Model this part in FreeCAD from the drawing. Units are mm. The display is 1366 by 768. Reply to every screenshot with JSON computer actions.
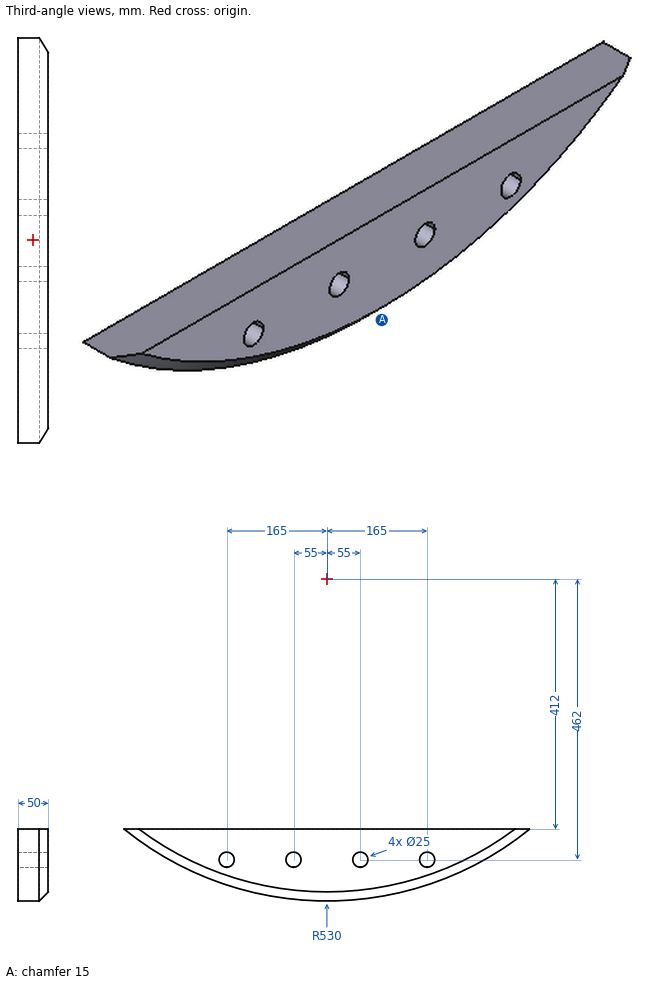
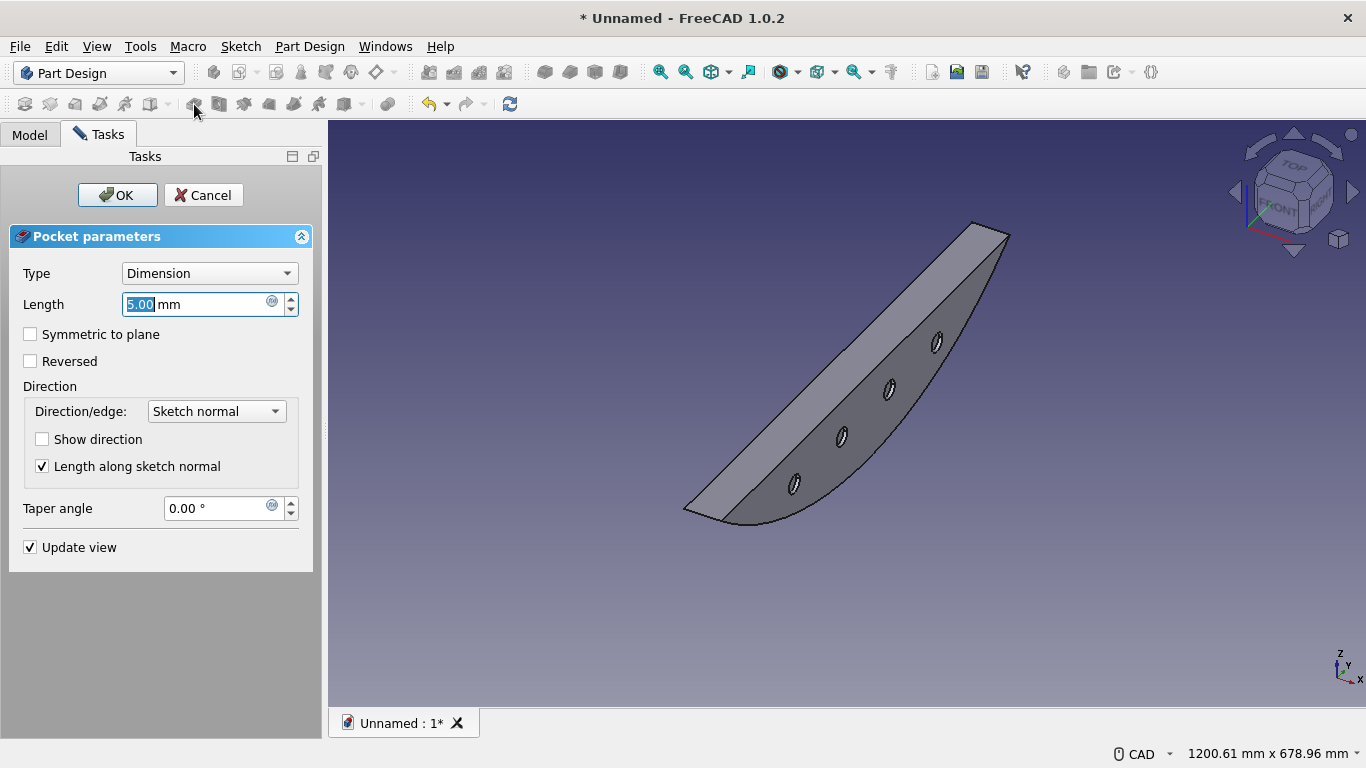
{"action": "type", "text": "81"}
{"action": "key", "text": "Tab"}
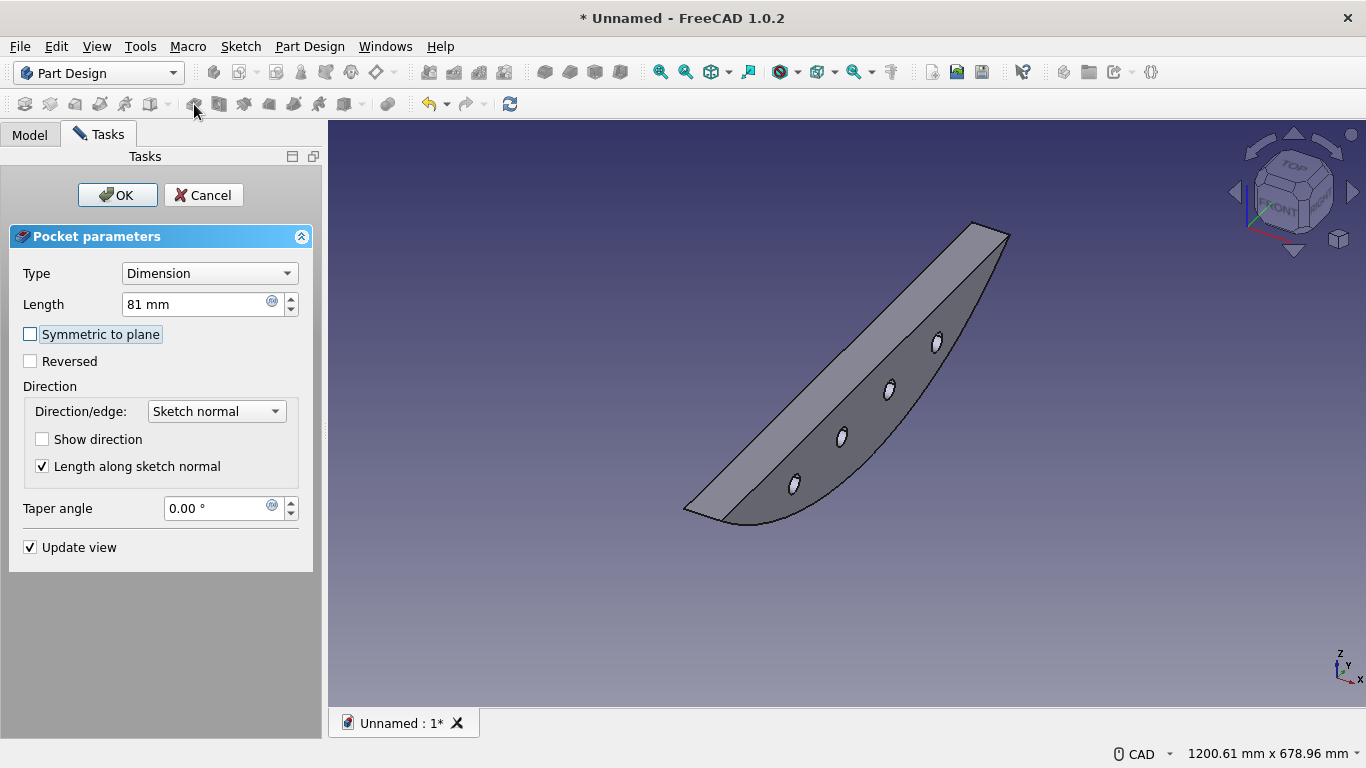
{"action": "left_click", "coordinate": [118, 195]}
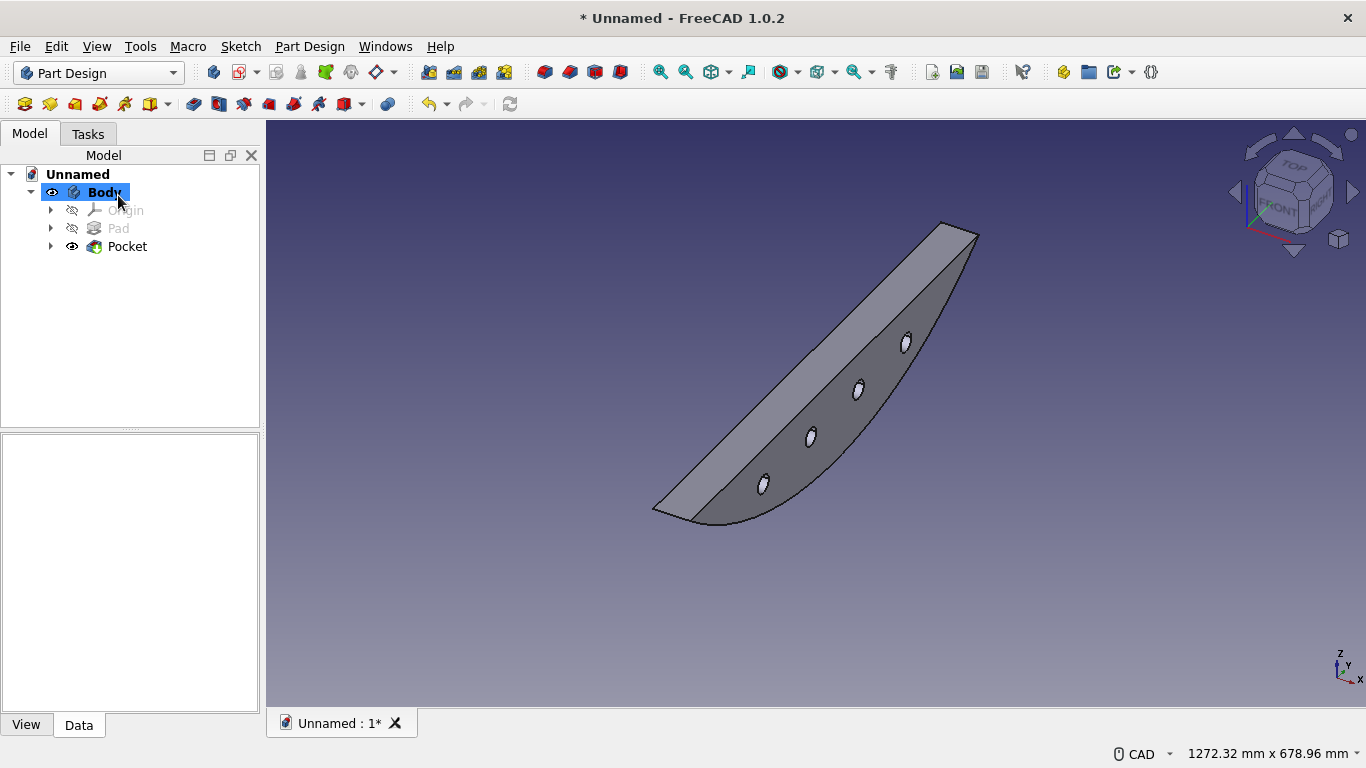
{"action": "key", "text": "0"}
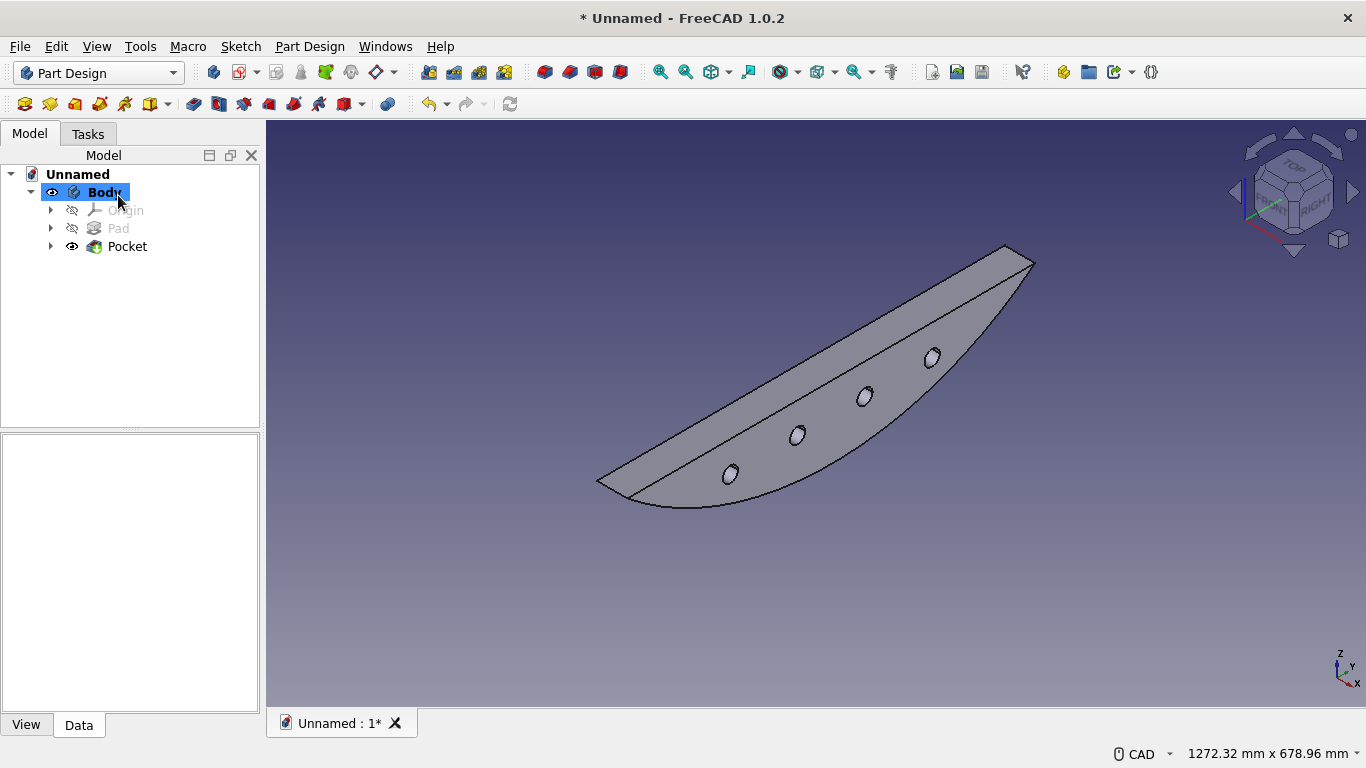
{"action": "key", "text": "2"}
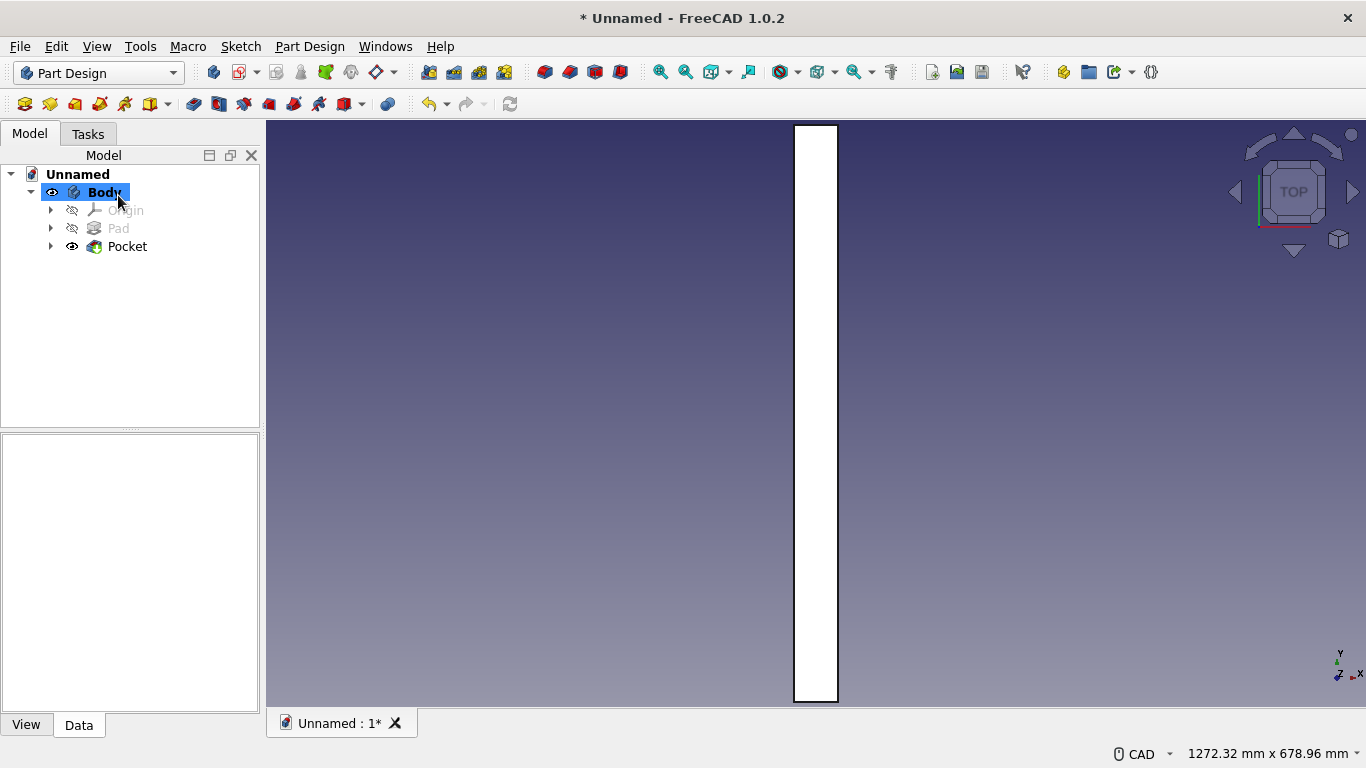
{"action": "key", "text": "1"}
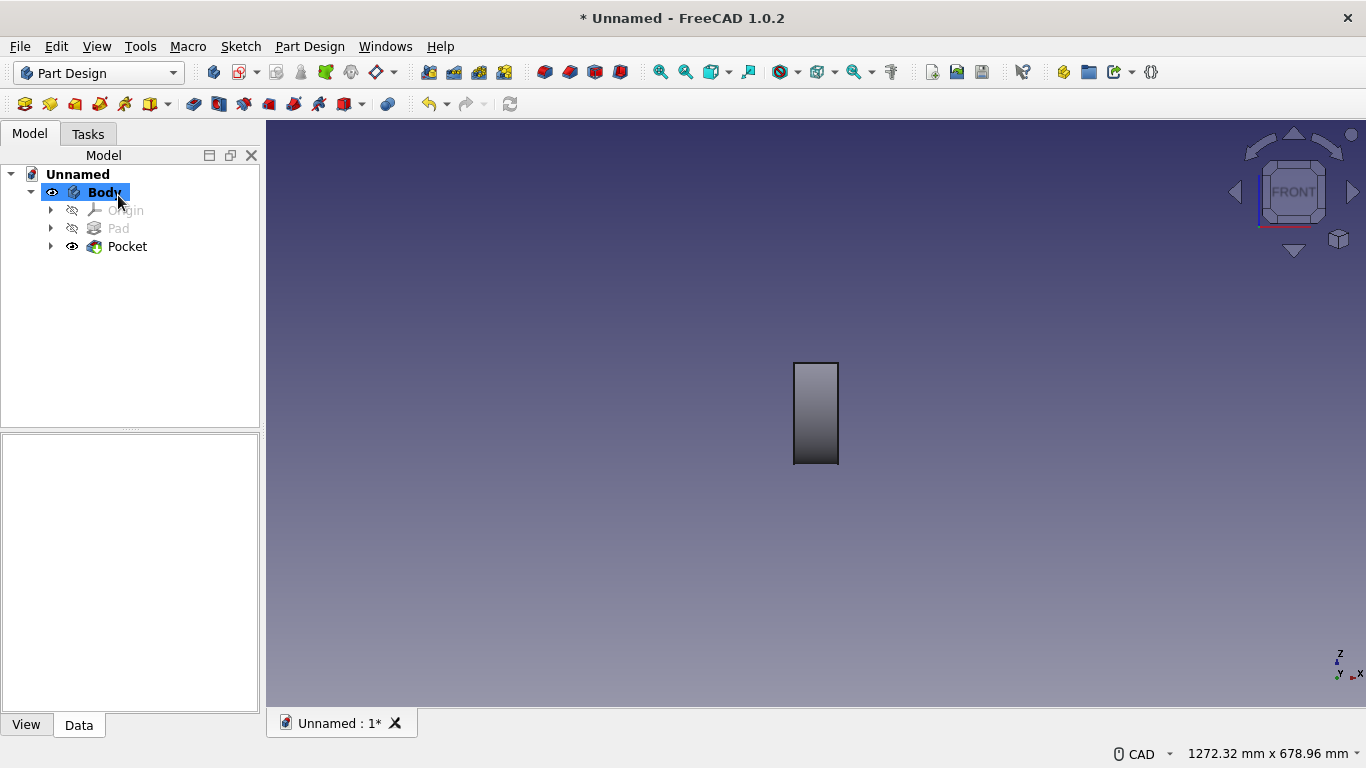
{"action": "left_click", "coordinate": [661, 72]}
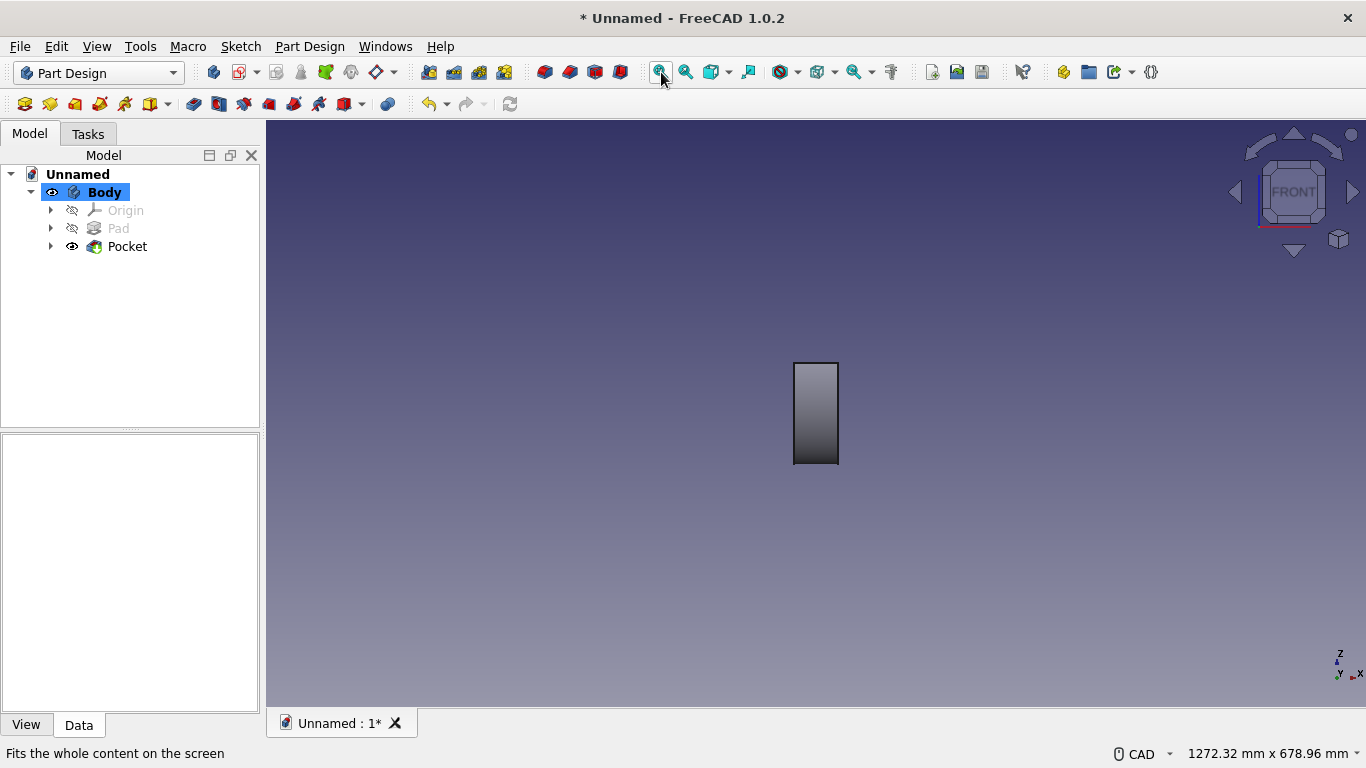
{"action": "left_click", "coordinate": [838, 459]}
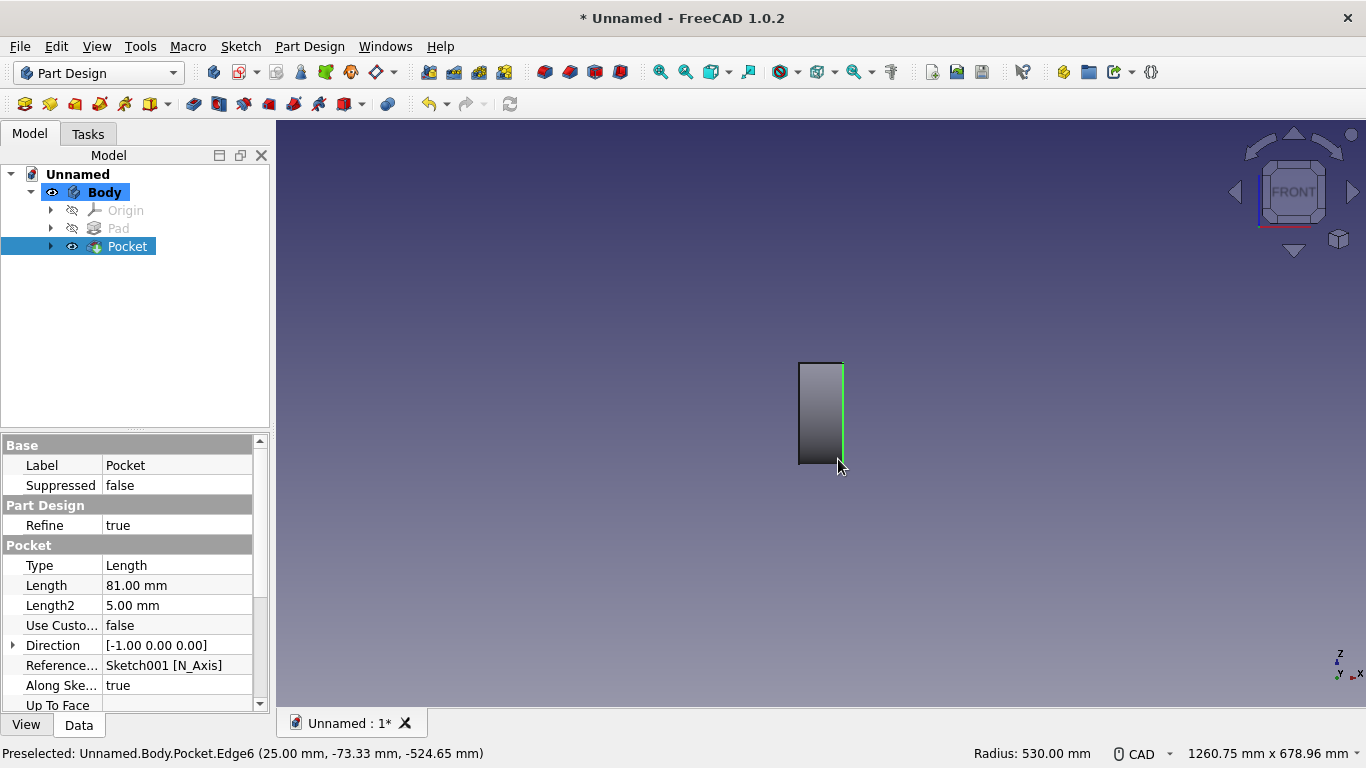
{"action": "left_click", "coordinate": [570, 72]}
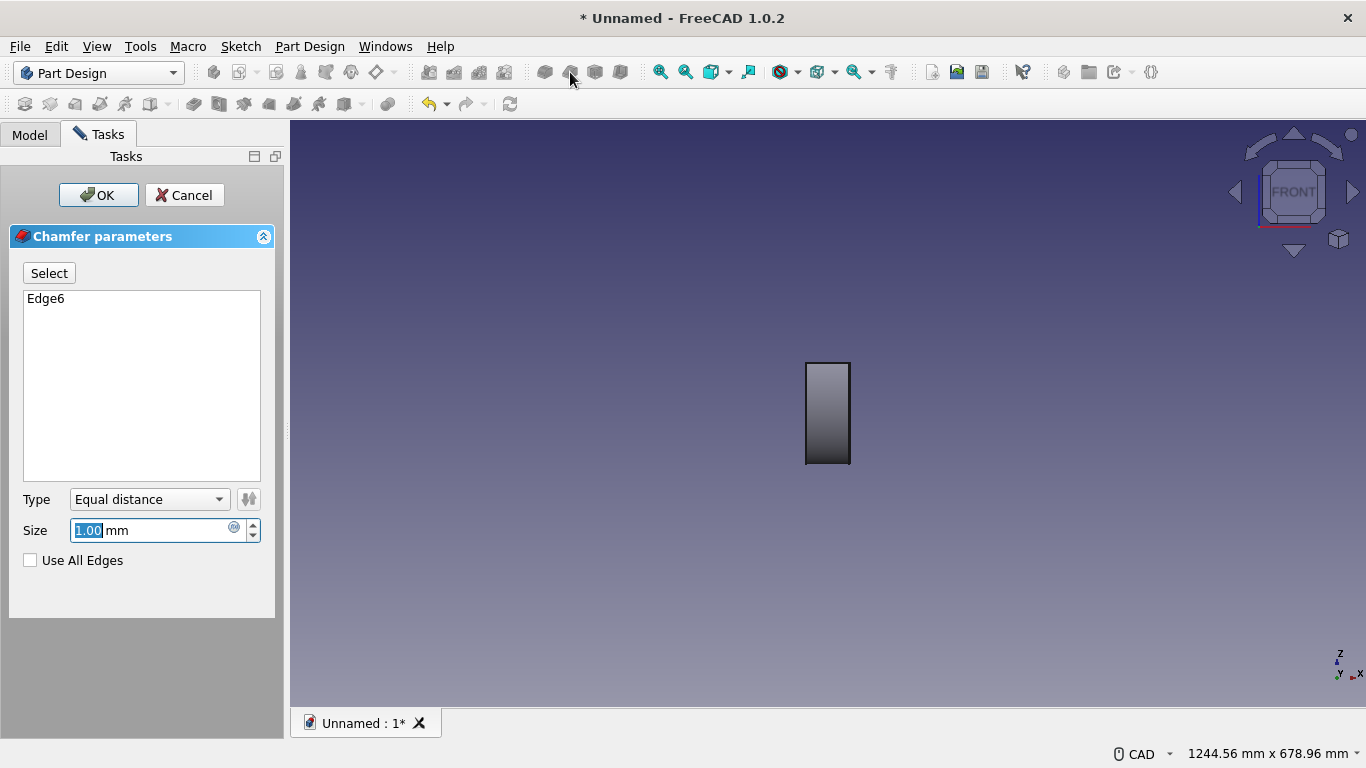
{"action": "type", "text": "15"}
{"action": "key", "text": "Tab"}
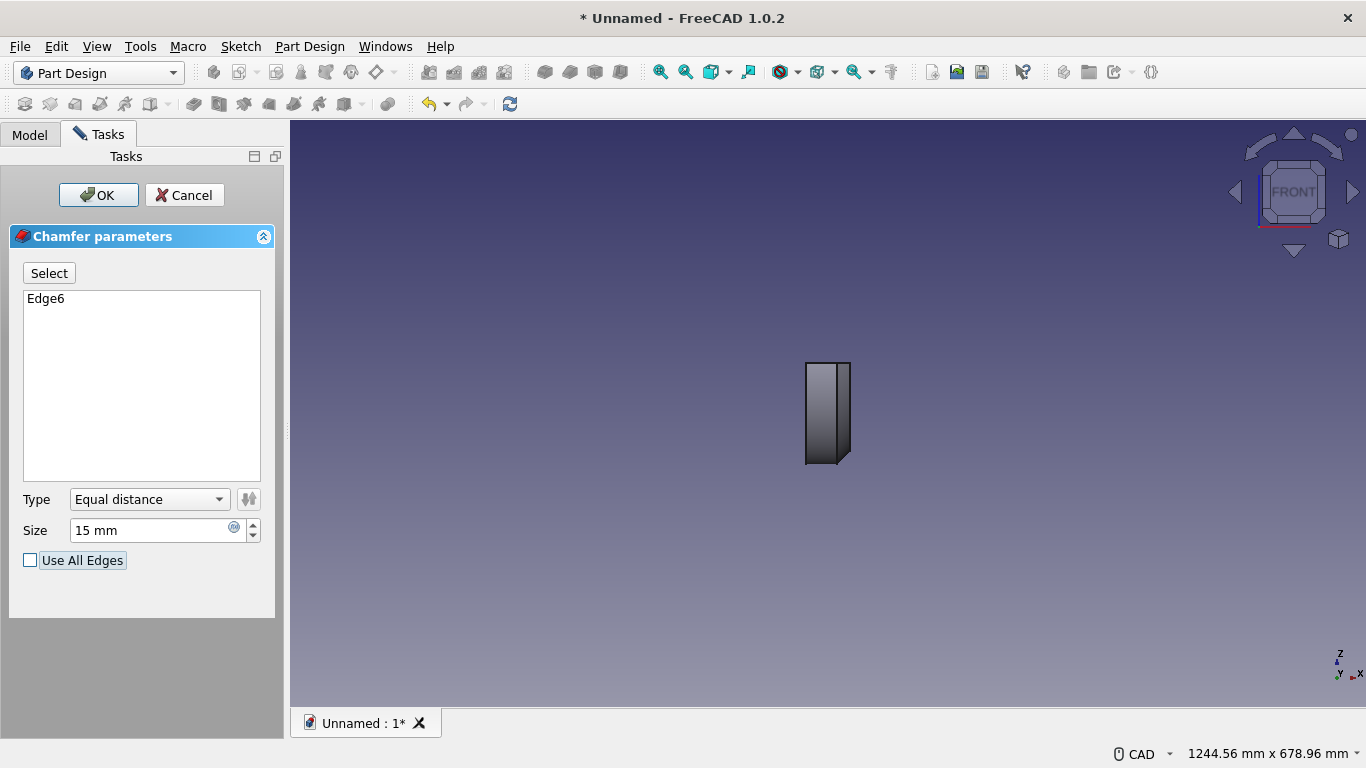
{"action": "left_click", "coordinate": [99, 195]}